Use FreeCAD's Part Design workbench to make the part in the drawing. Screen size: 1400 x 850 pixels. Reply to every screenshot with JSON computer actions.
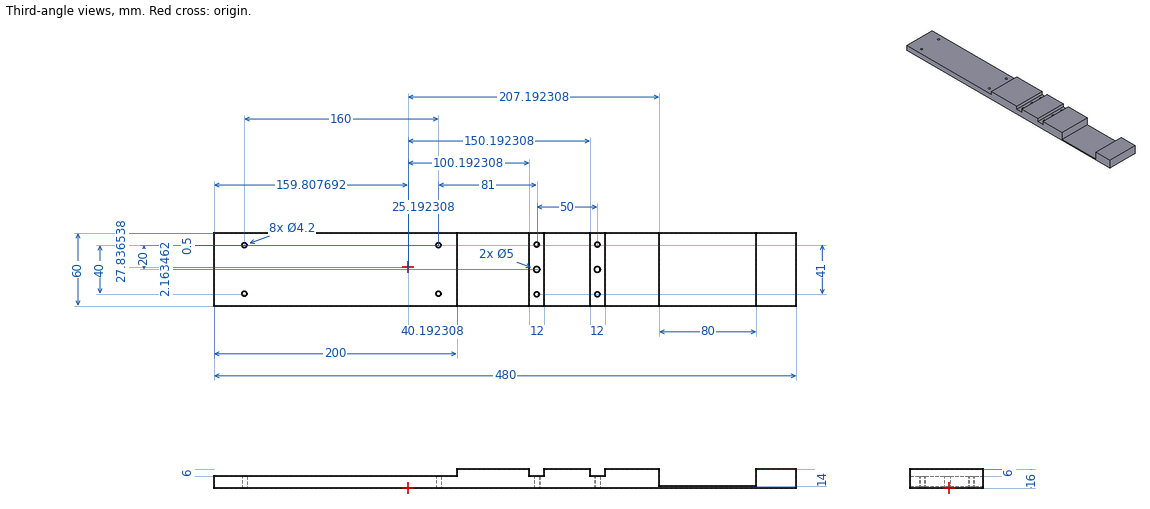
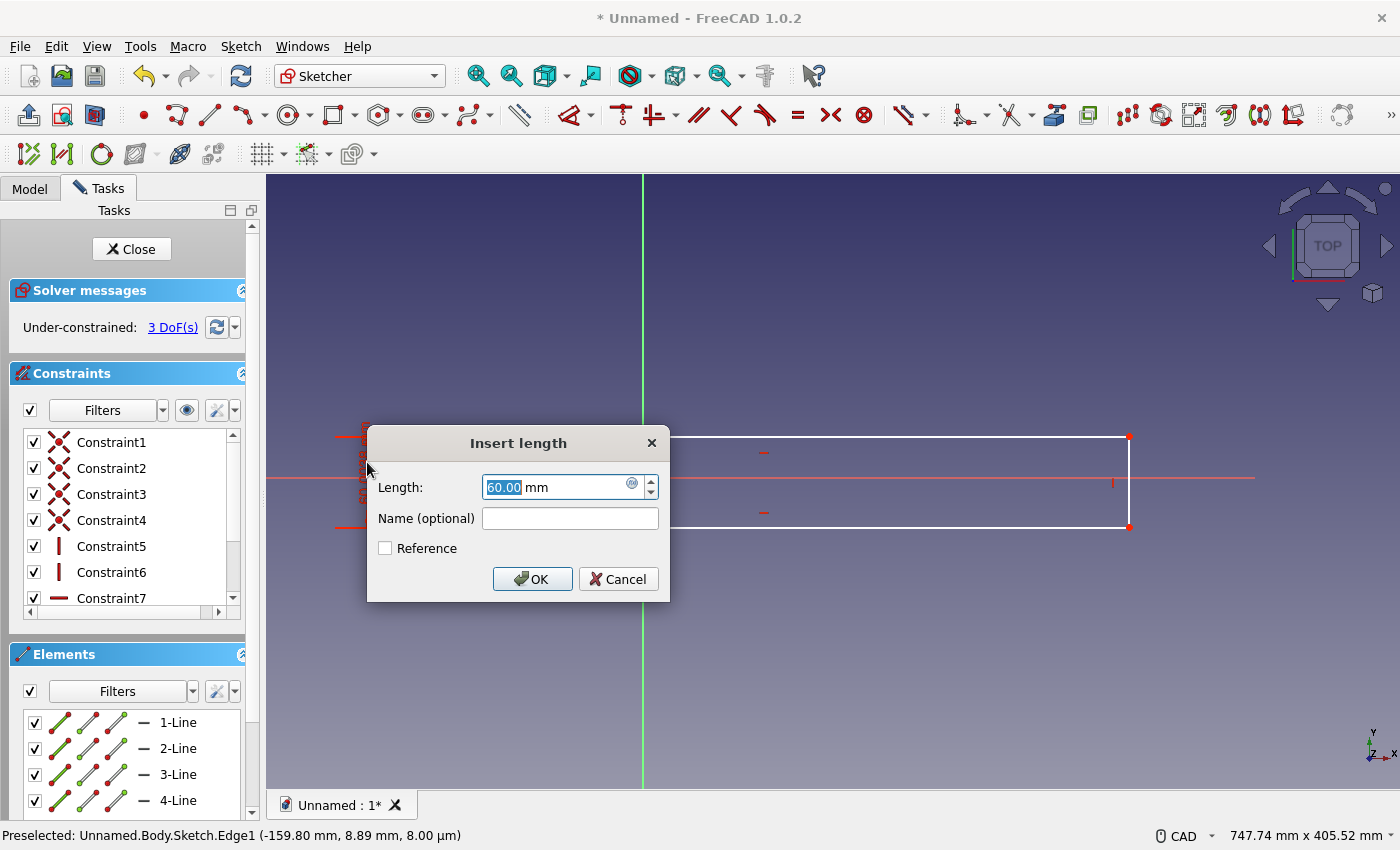
{"action": "type", "text": "60"}
{"action": "key", "text": "Return"}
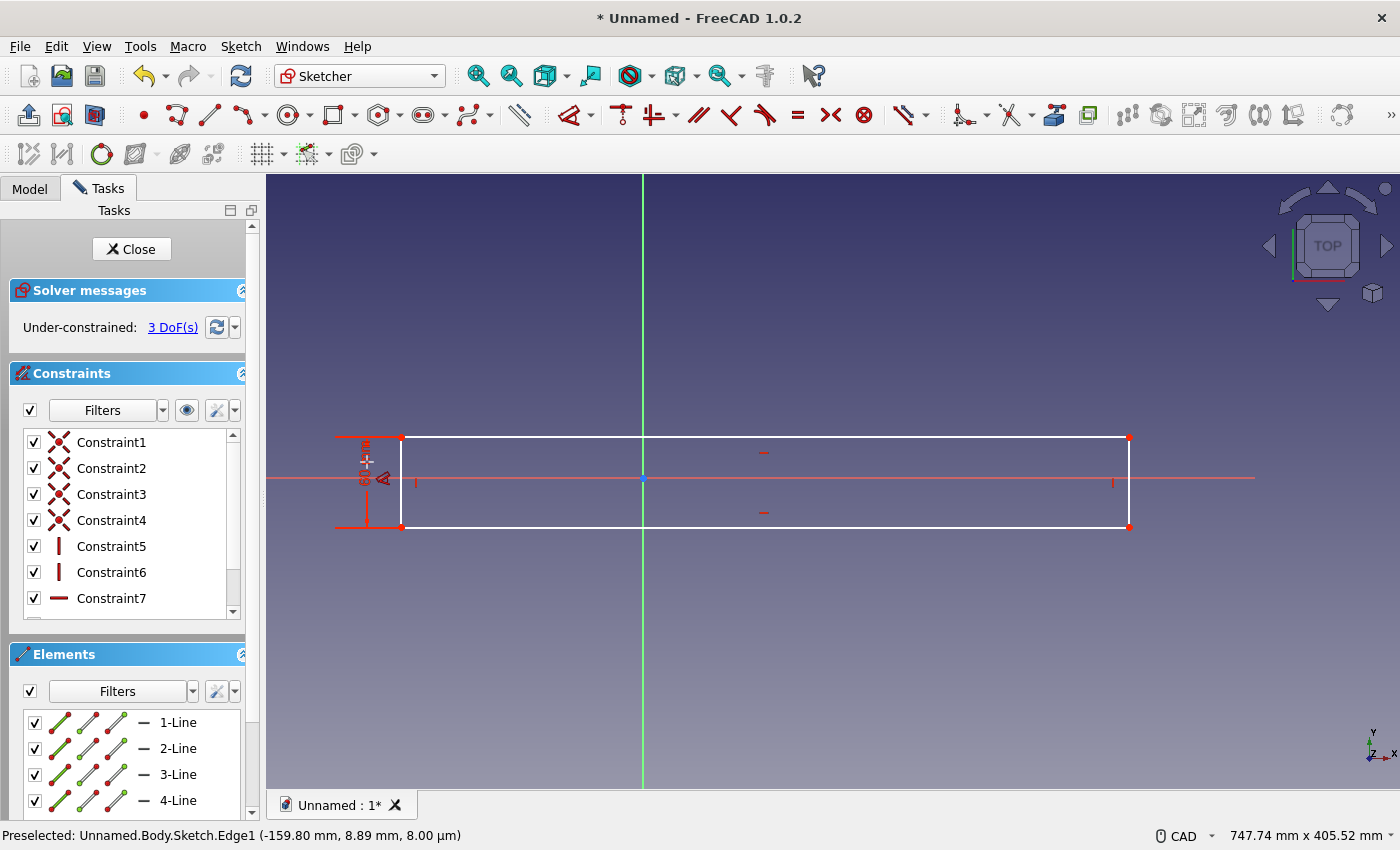
{"action": "left_click", "coordinate": [619, 528]}
{"action": "left_click", "coordinate": [765, 562]}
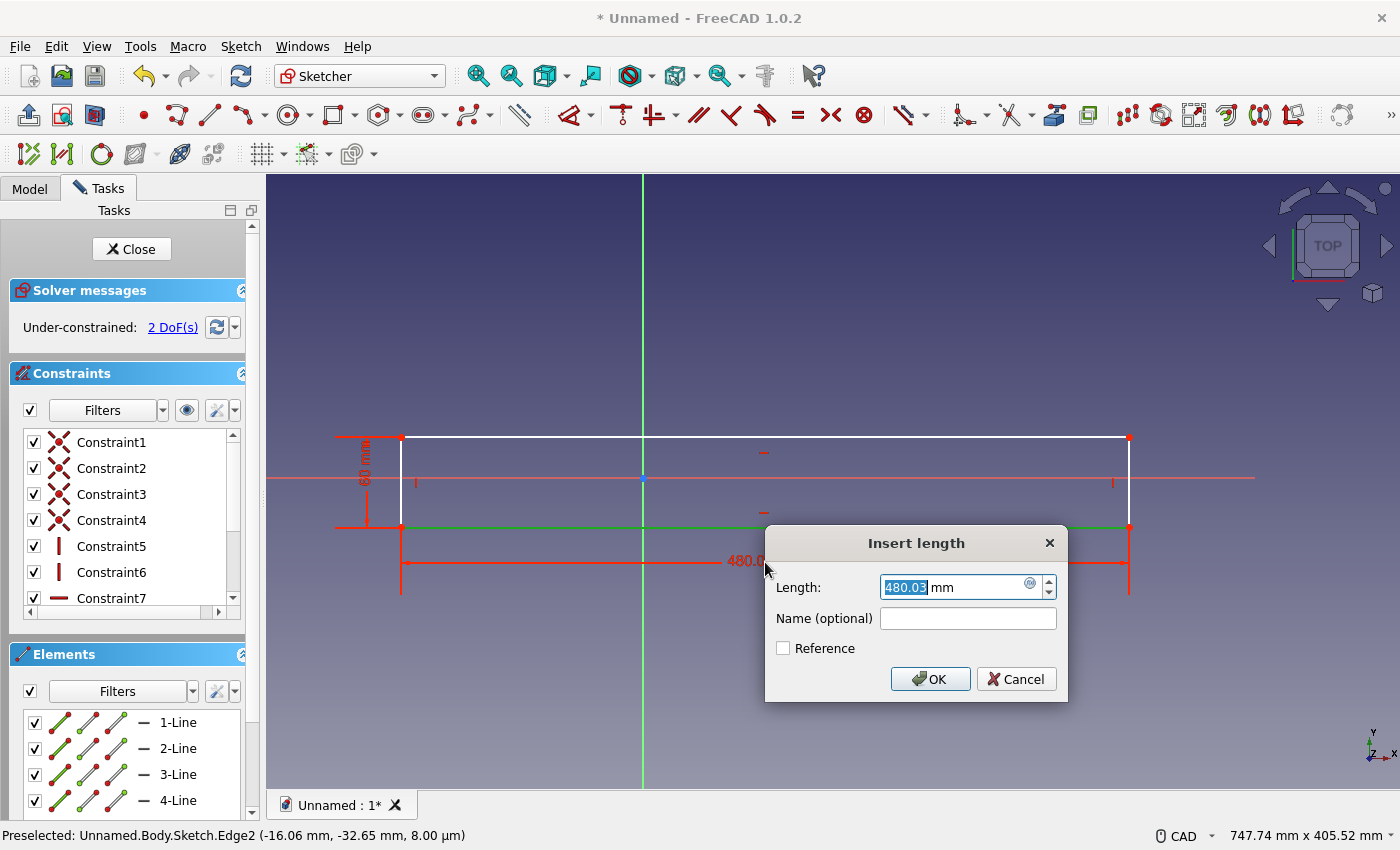
{"action": "type", "text": "480"}
{"action": "key", "text": "Return"}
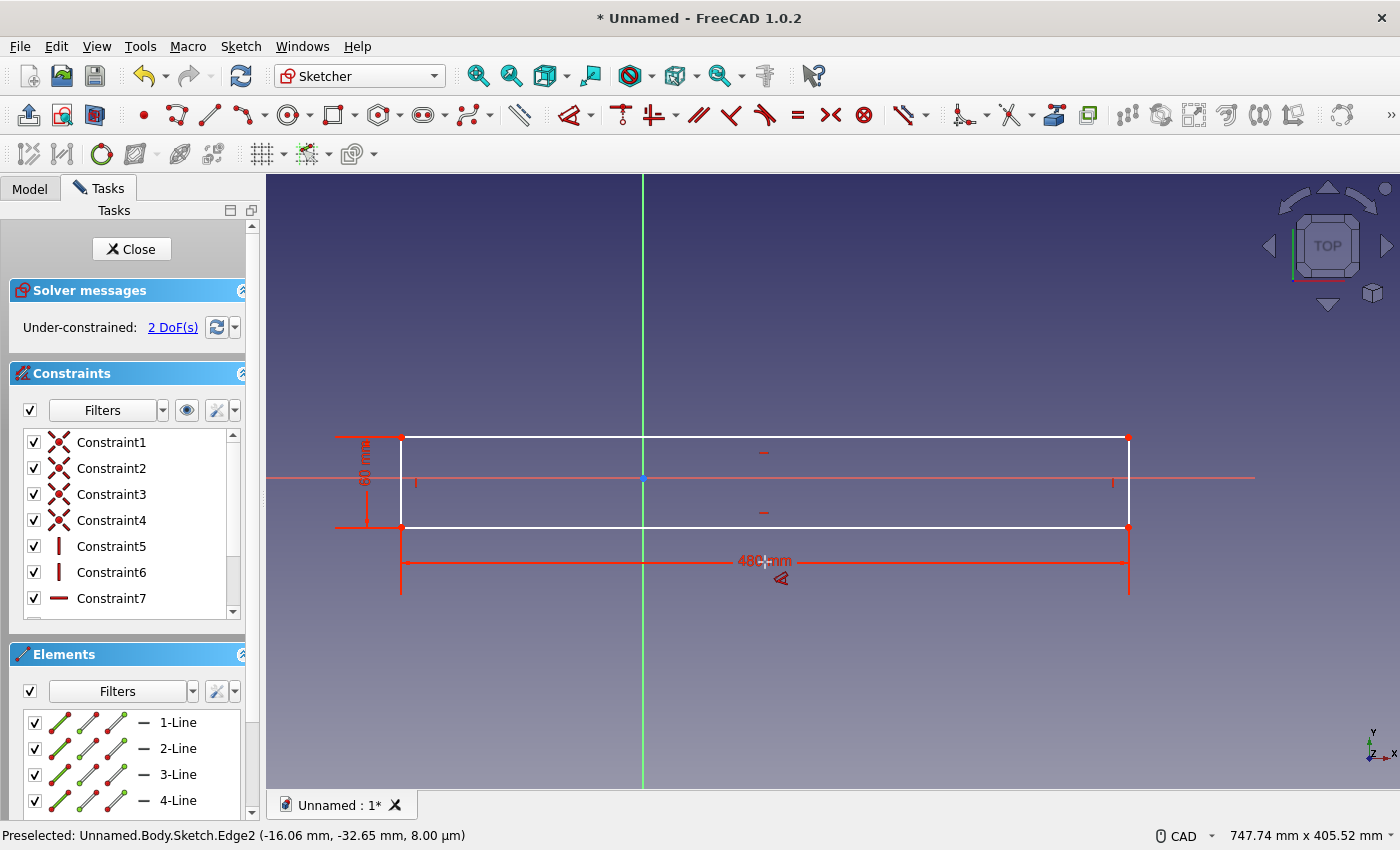
{"action": "left_click", "coordinate": [401, 437]}
{"action": "left_click", "coordinate": [677, 458]}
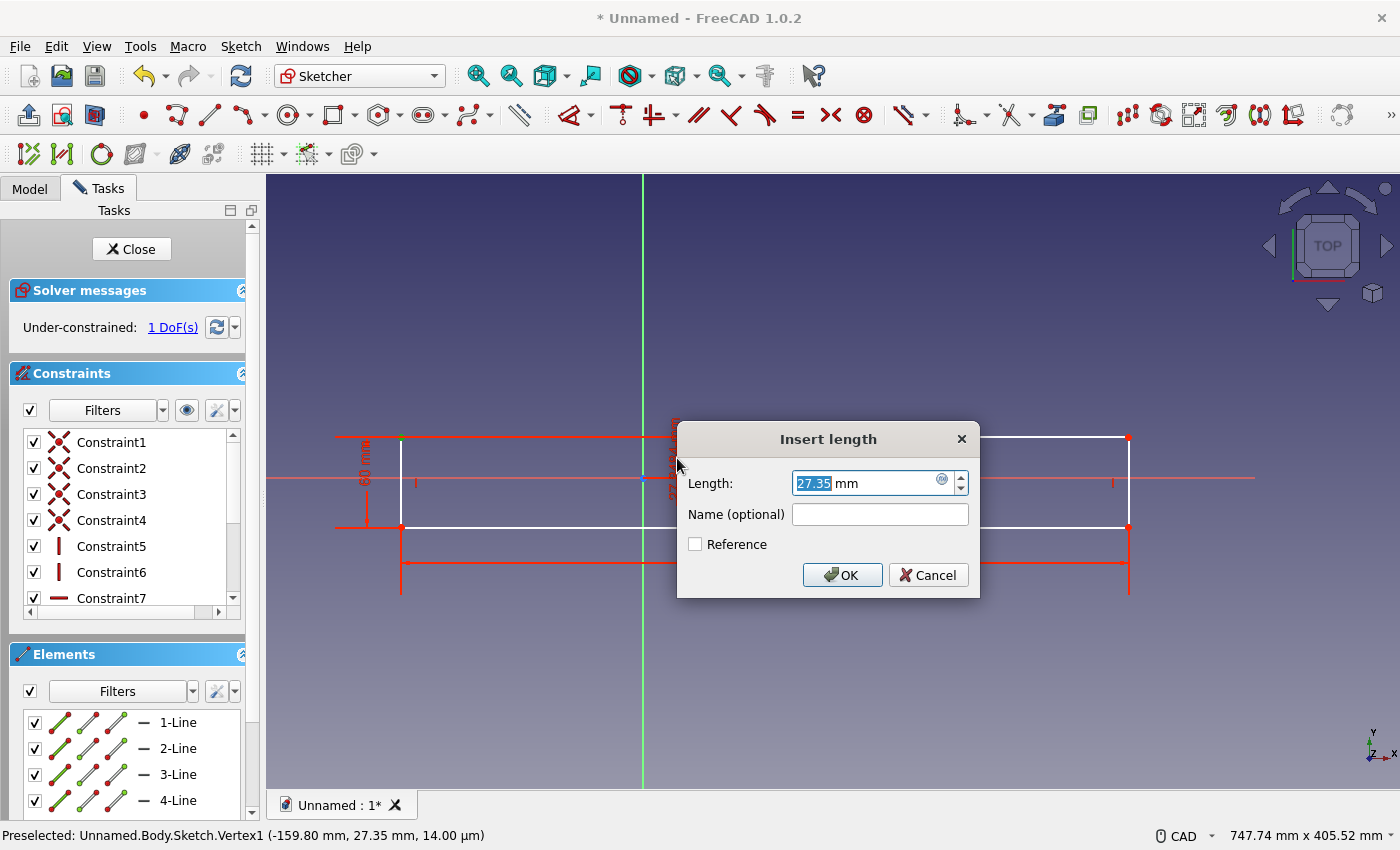
{"action": "type", "text": "27.836538"}
{"action": "key", "text": "Return"}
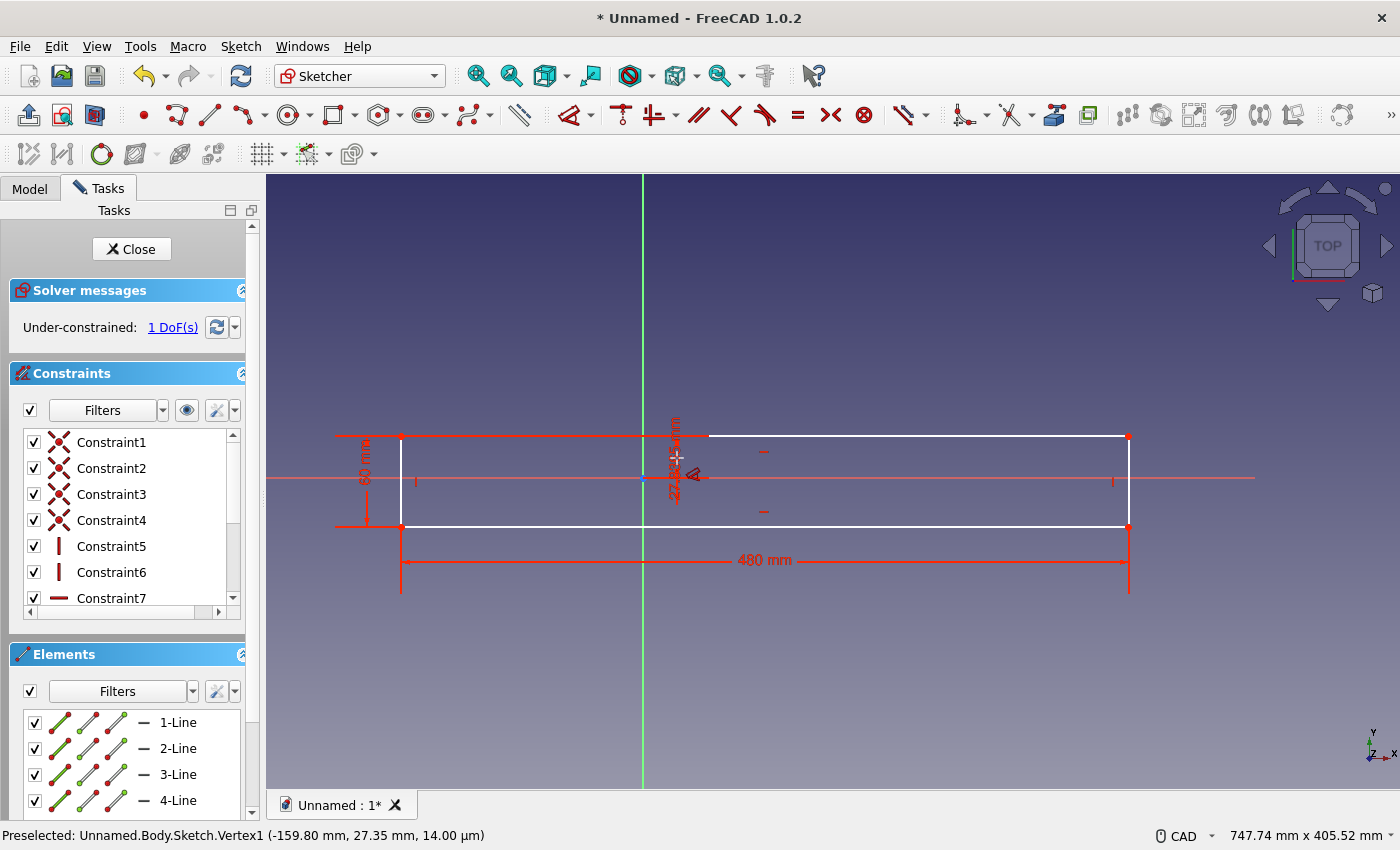
{"action": "left_click", "coordinate": [401, 436]}
{"action": "left_click", "coordinate": [522, 402]}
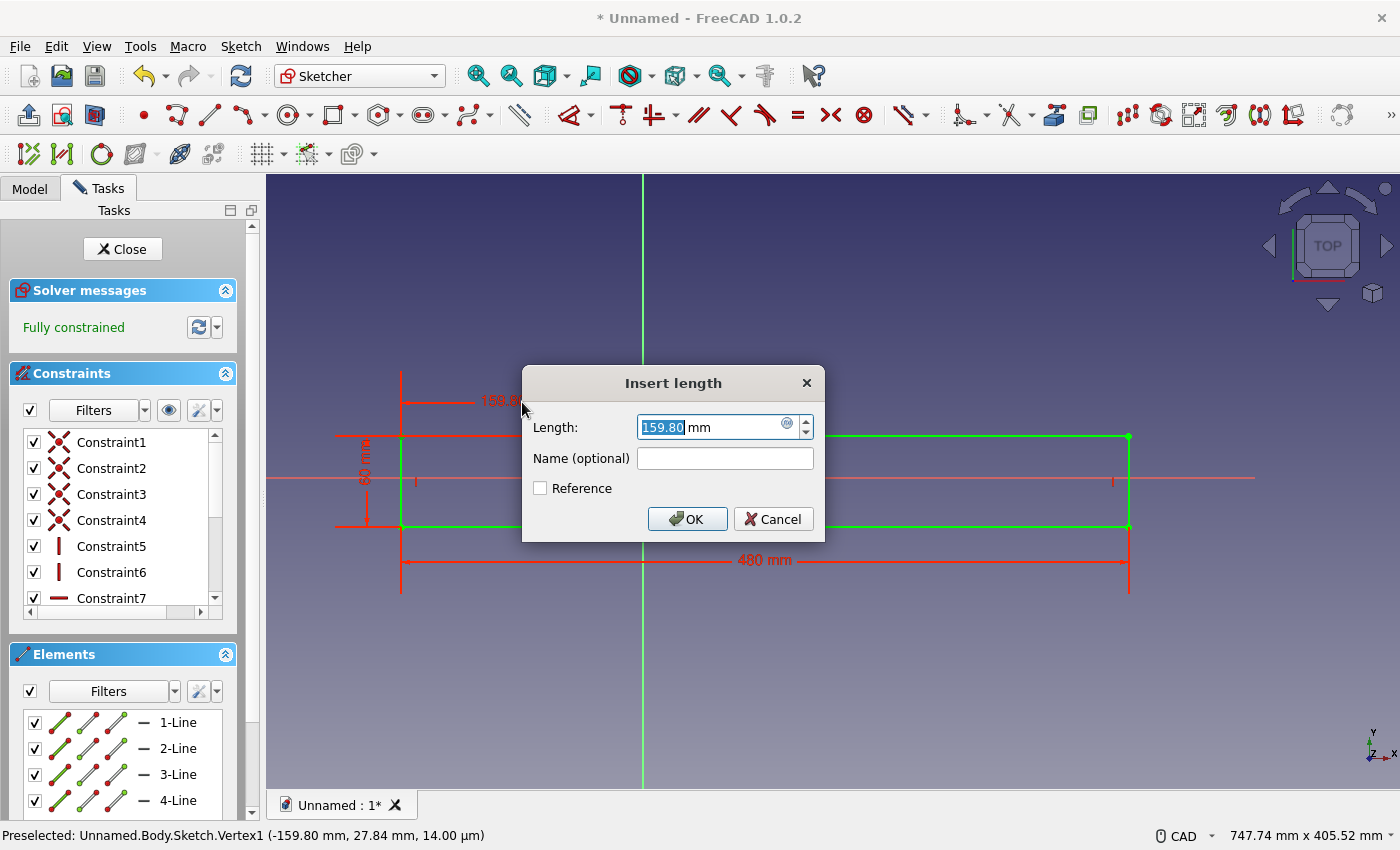
{"action": "type", "text": "159.807692"}
{"action": "key", "text": "Return"}
{"action": "key", "text": "Escape"}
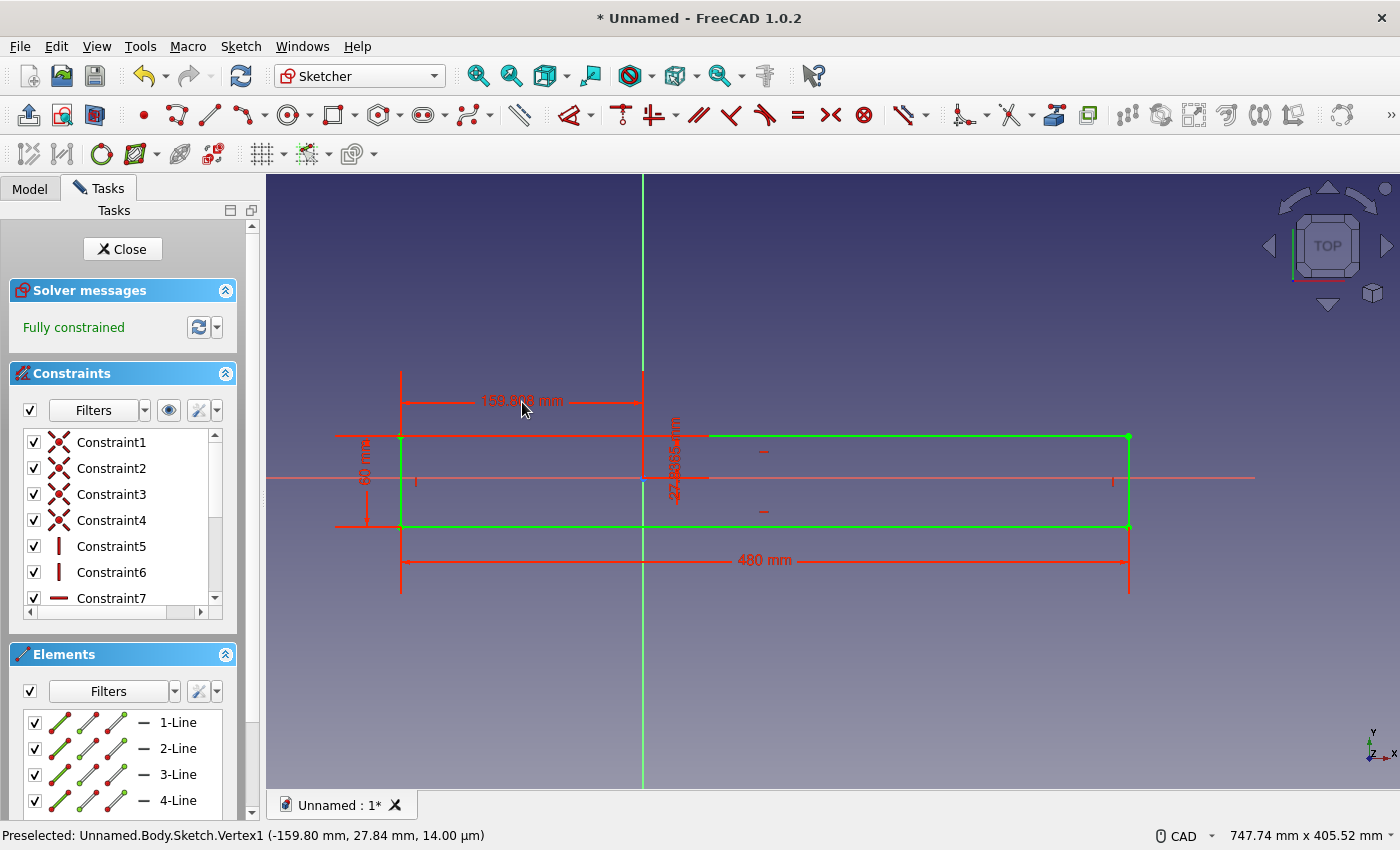
{"action": "left_click", "coordinate": [123, 249]}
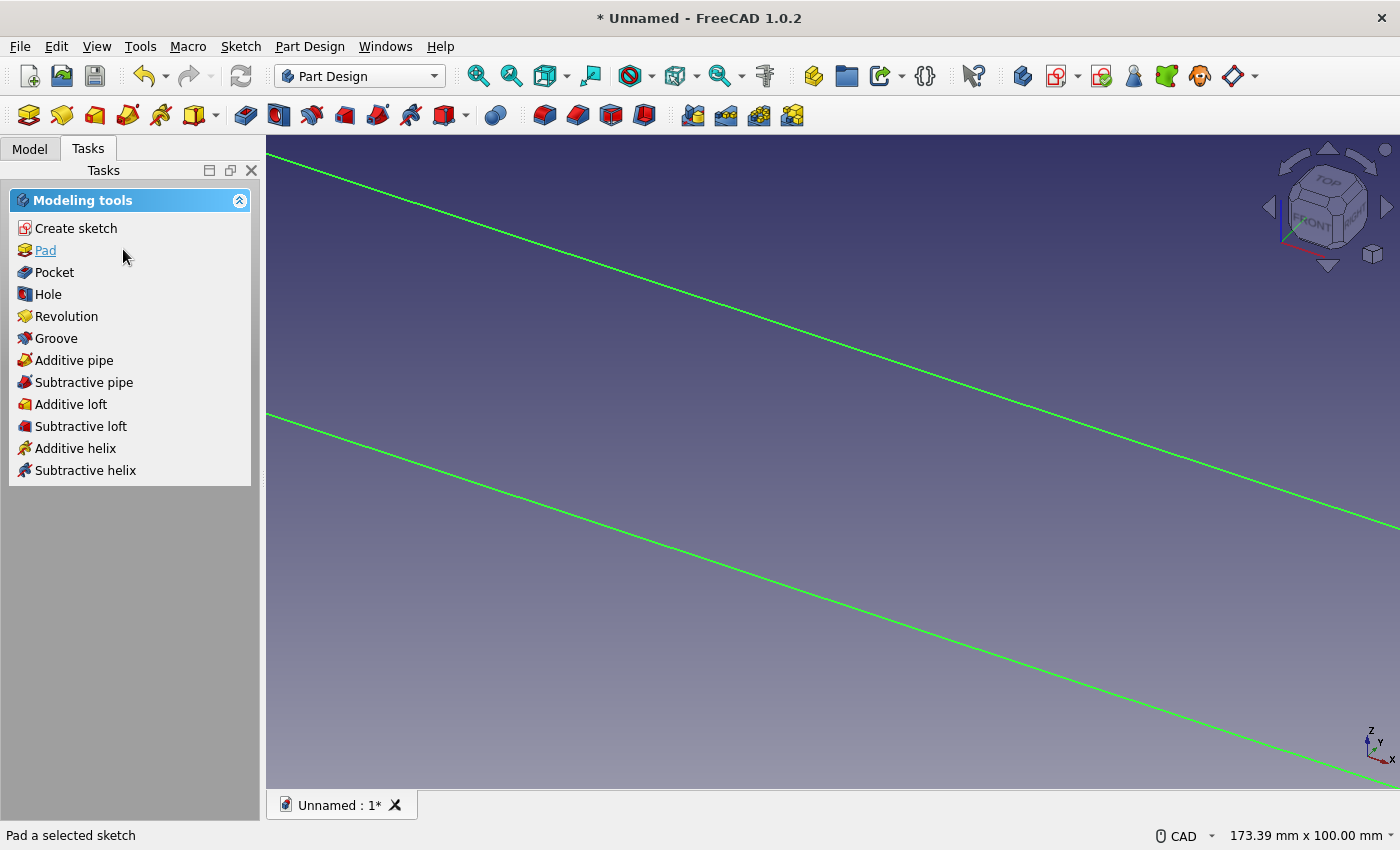
{"action": "left_click", "coordinate": [29, 116]}